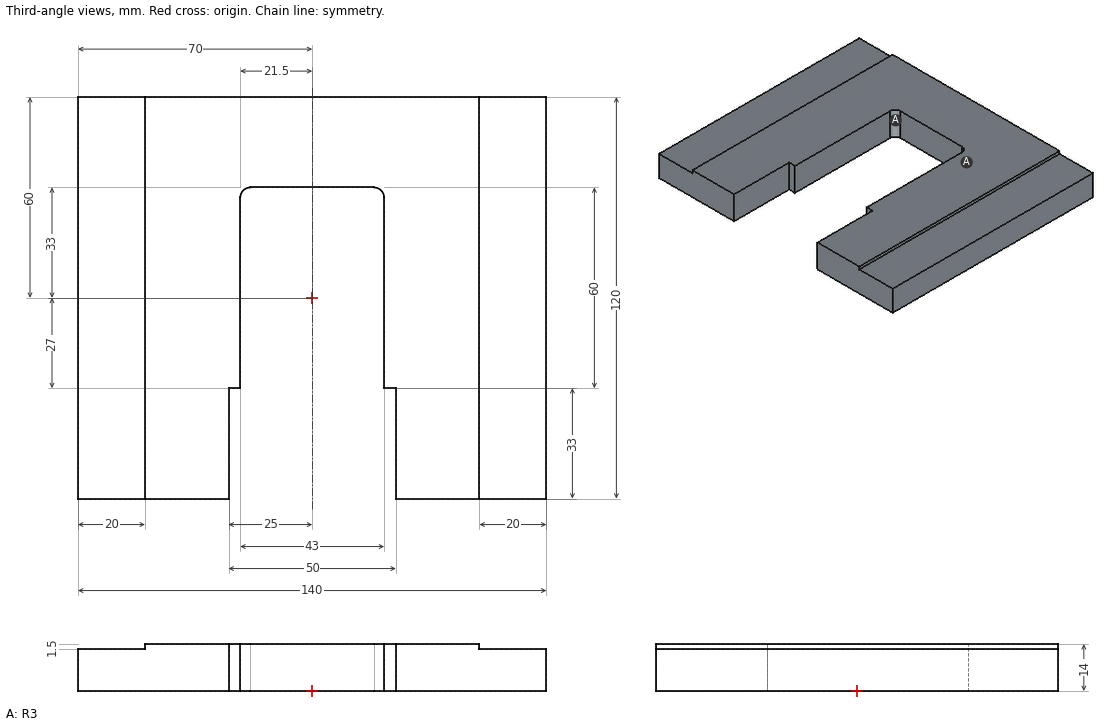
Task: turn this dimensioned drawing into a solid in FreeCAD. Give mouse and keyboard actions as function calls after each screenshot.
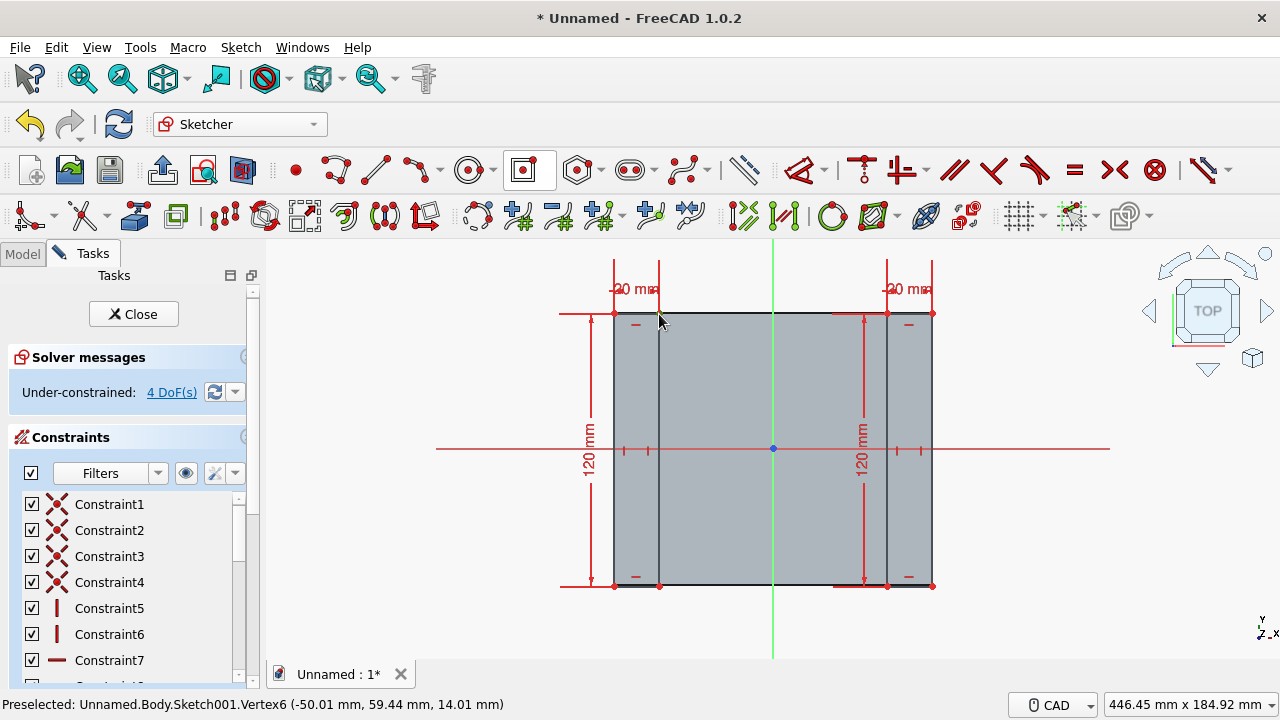
click(887, 314)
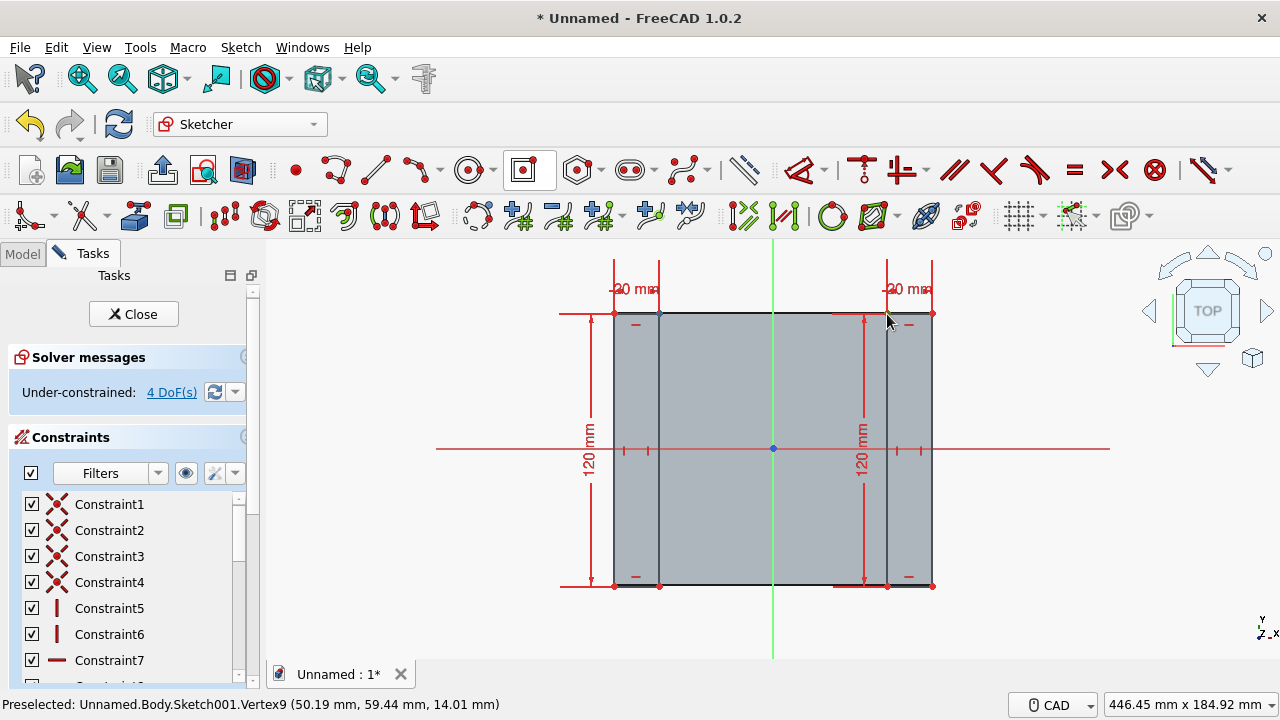
click(773, 605)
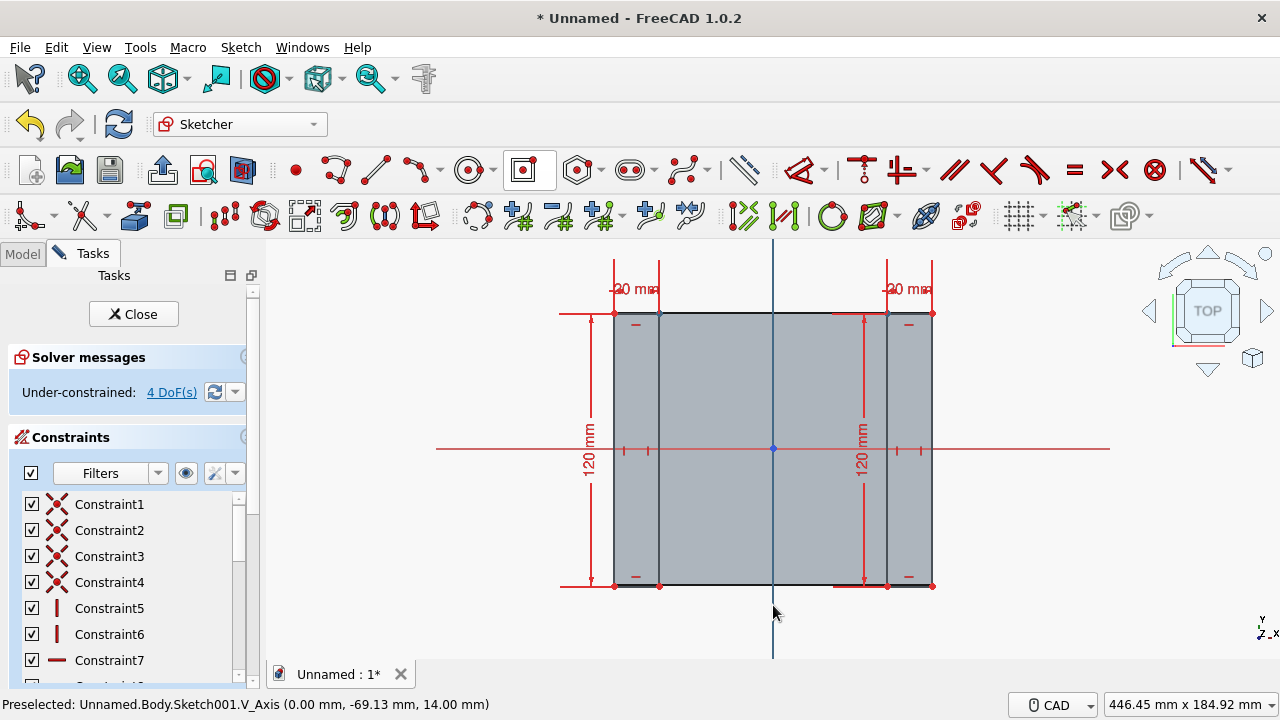
click(1116, 170)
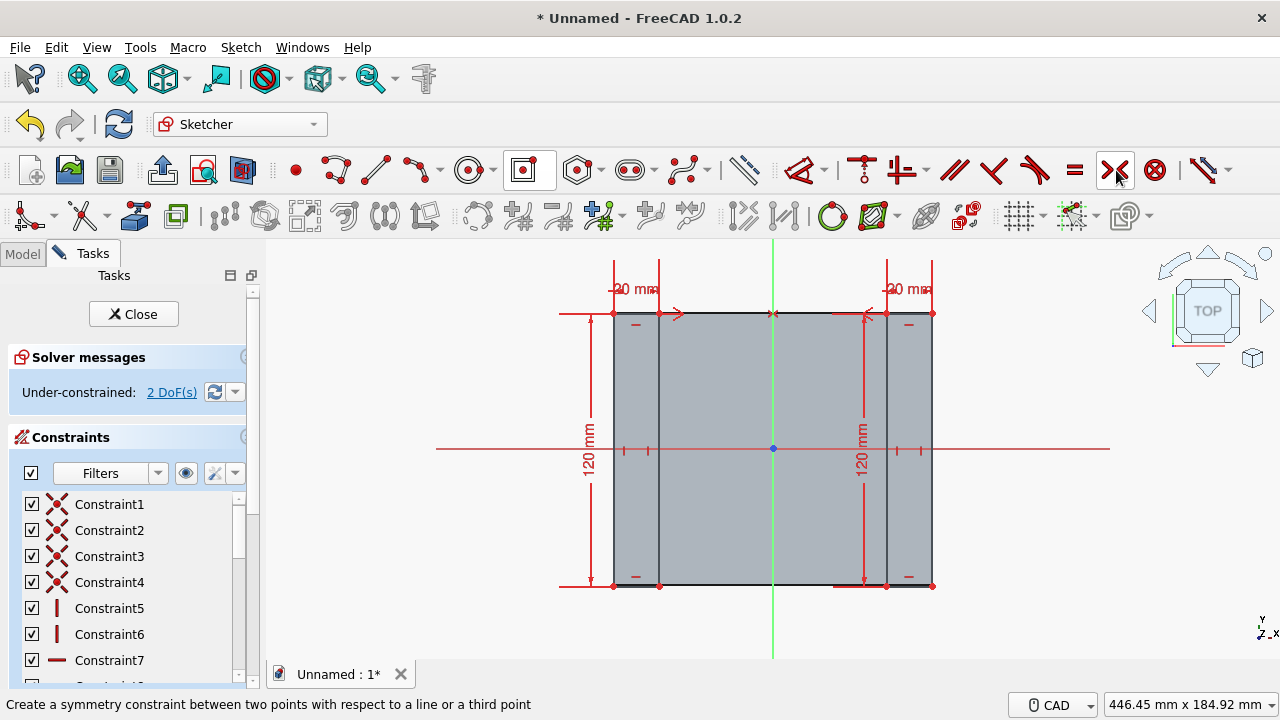
click(614, 314)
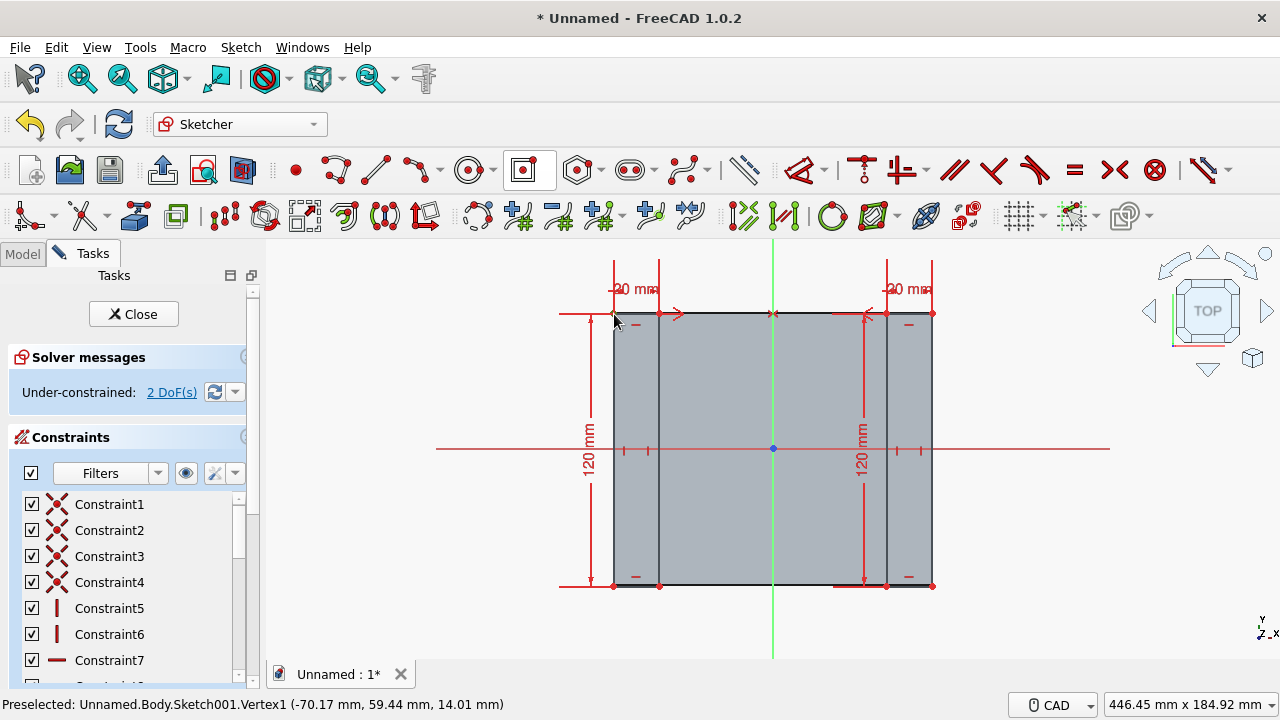
click(826, 170)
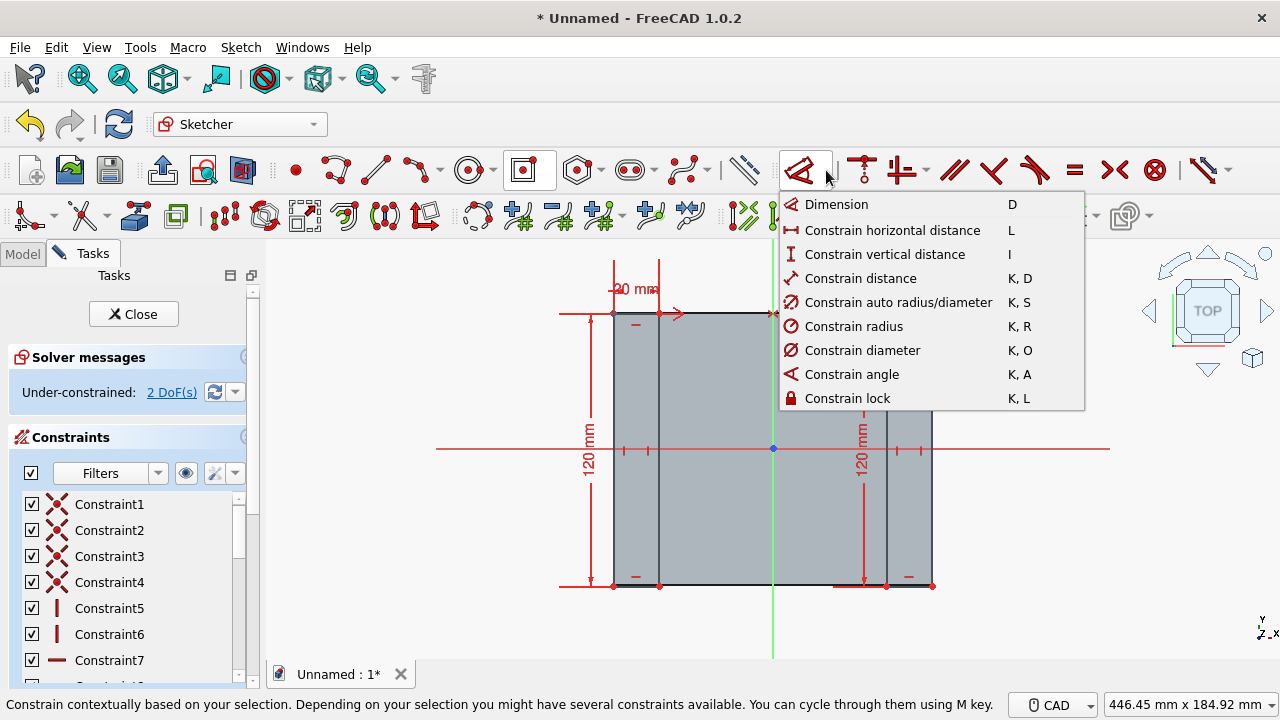
click(932, 230)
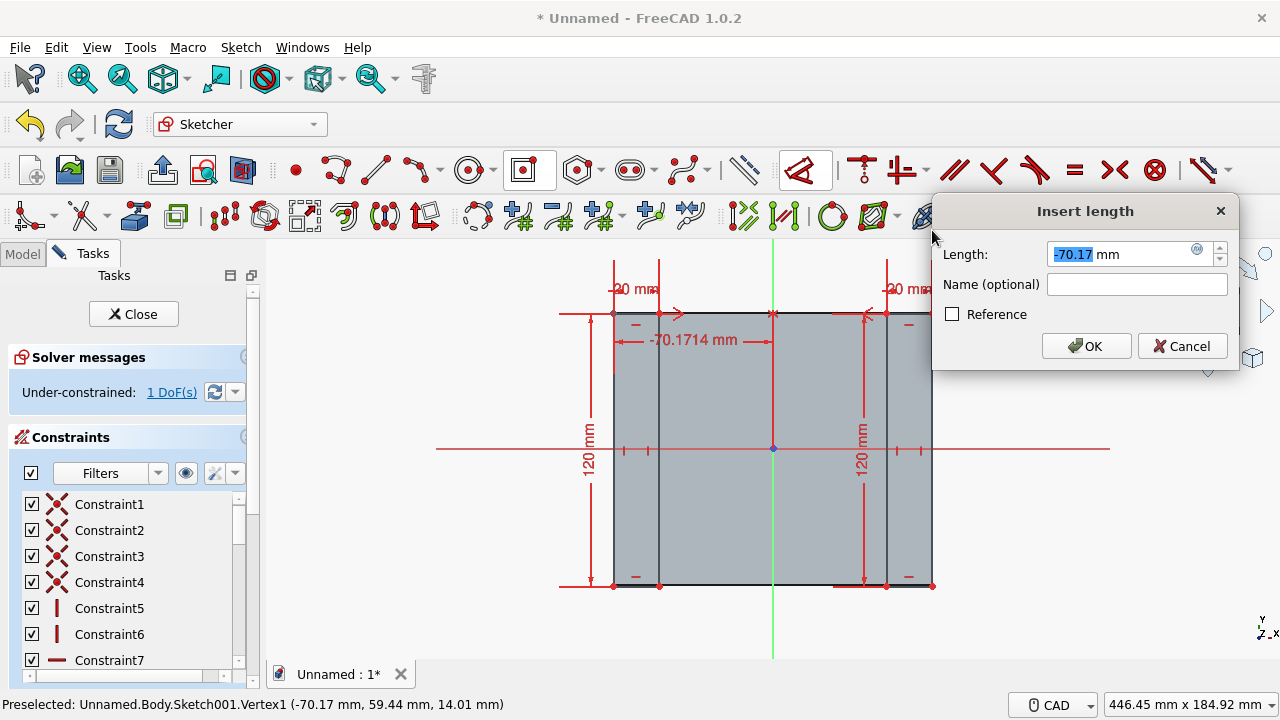
text(-70)
key(Return)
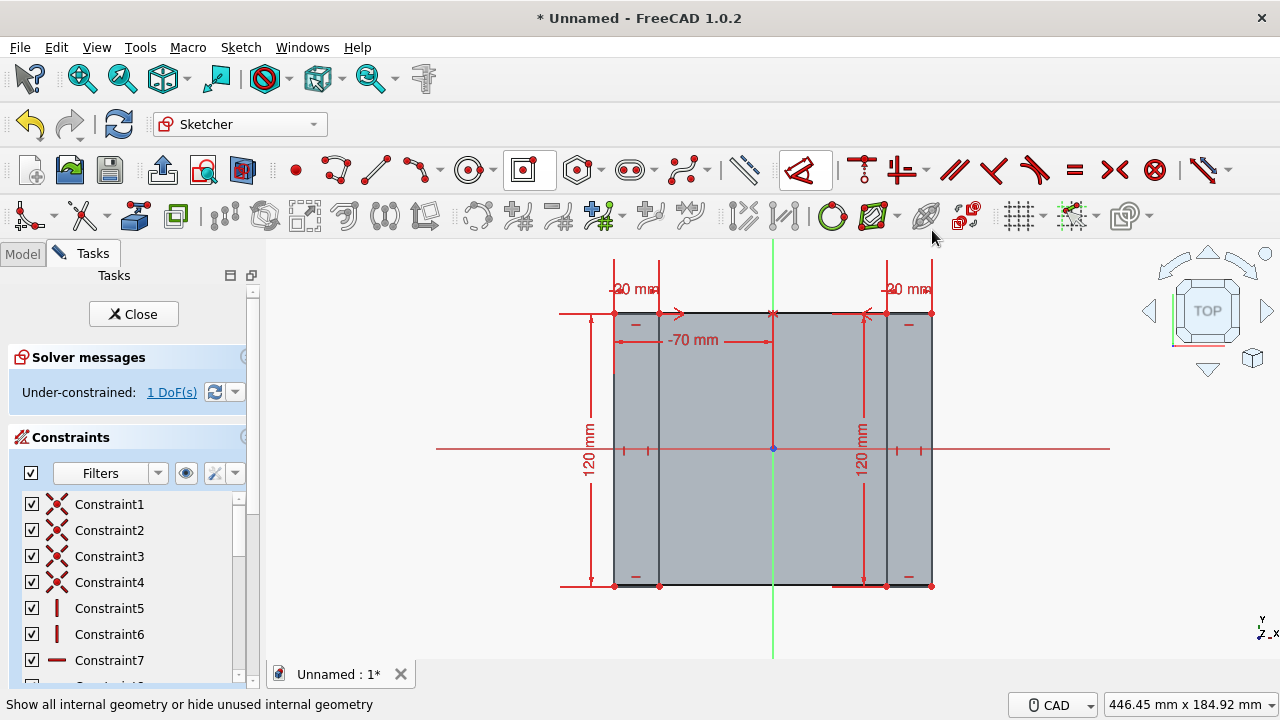
click(614, 314)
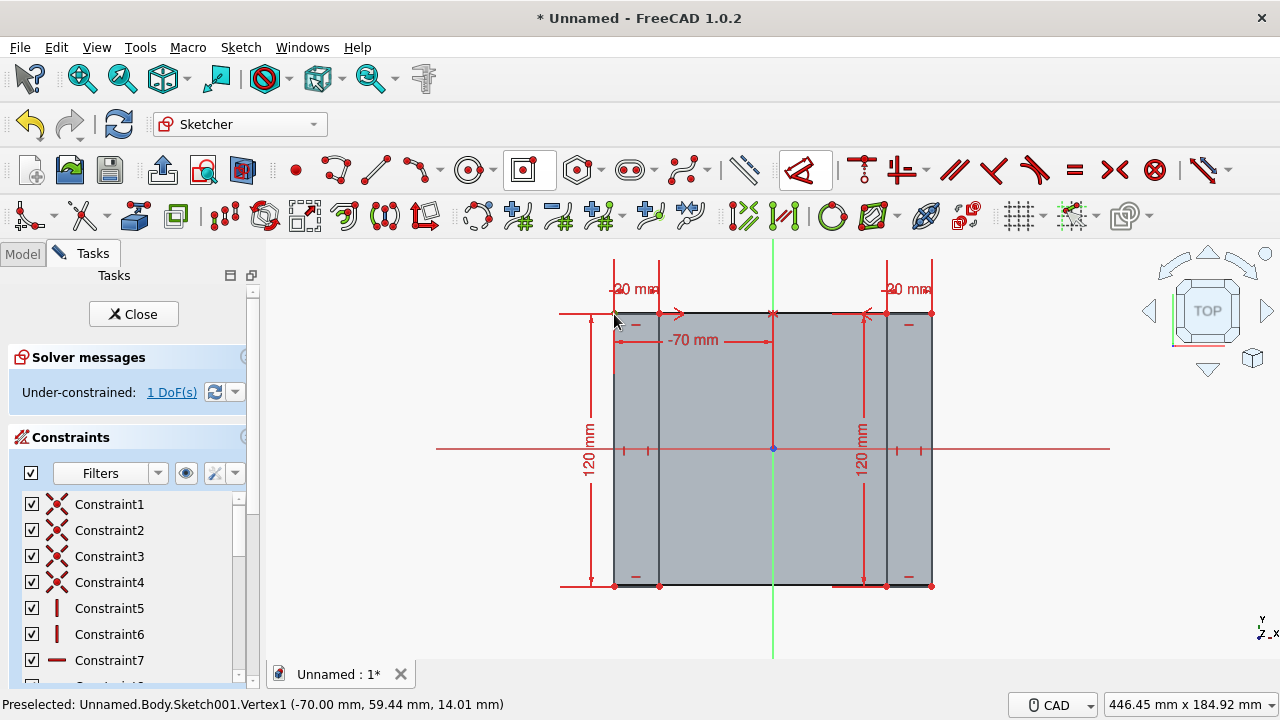
click(826, 170)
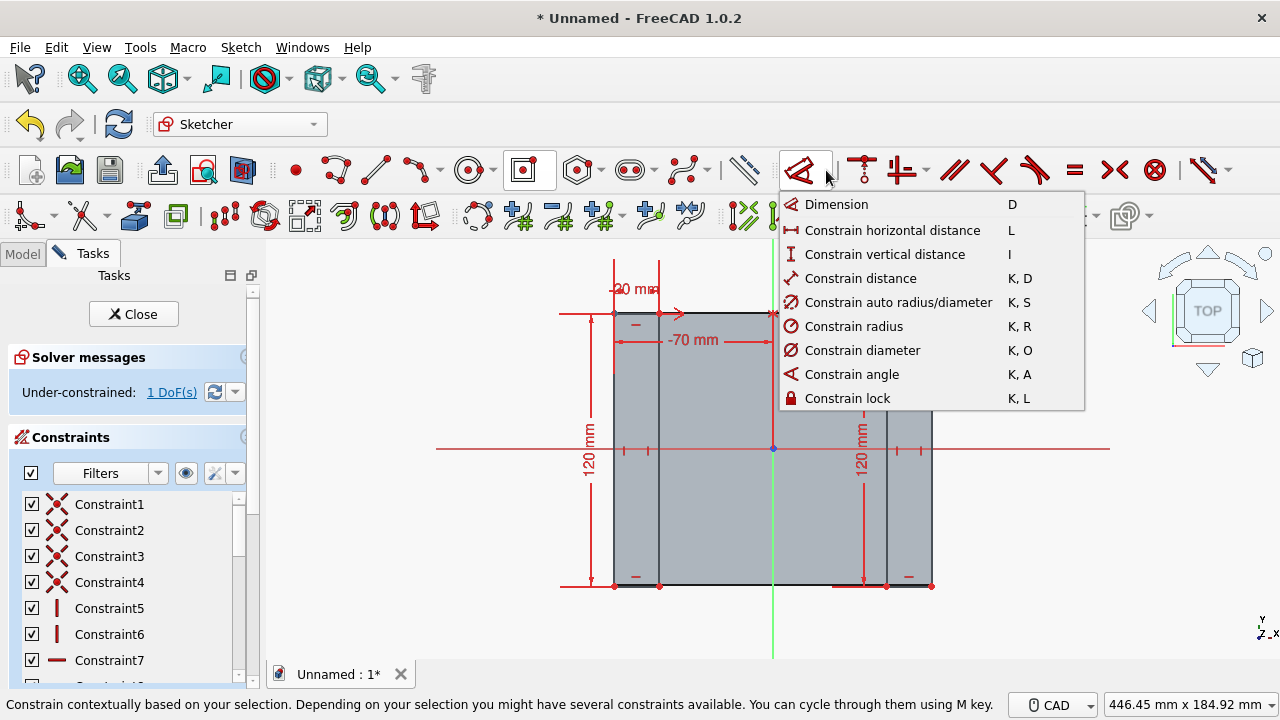
click(932, 254)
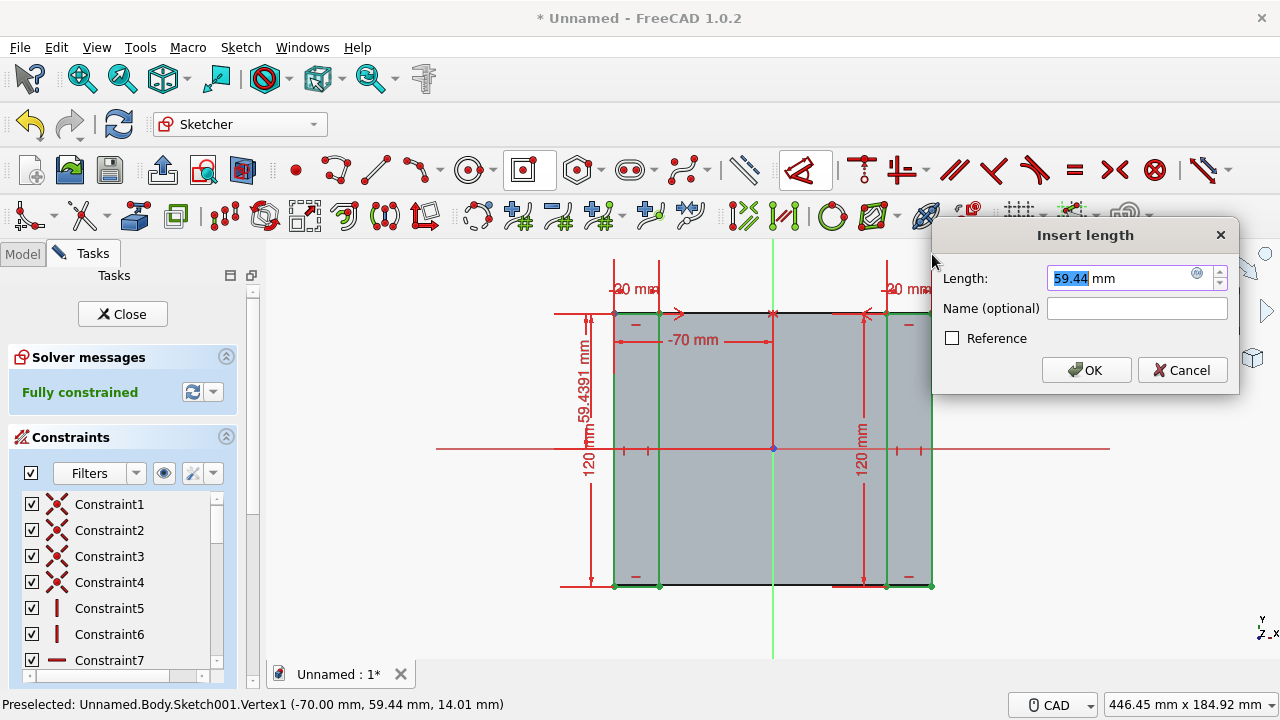
text(60)
key(Return)